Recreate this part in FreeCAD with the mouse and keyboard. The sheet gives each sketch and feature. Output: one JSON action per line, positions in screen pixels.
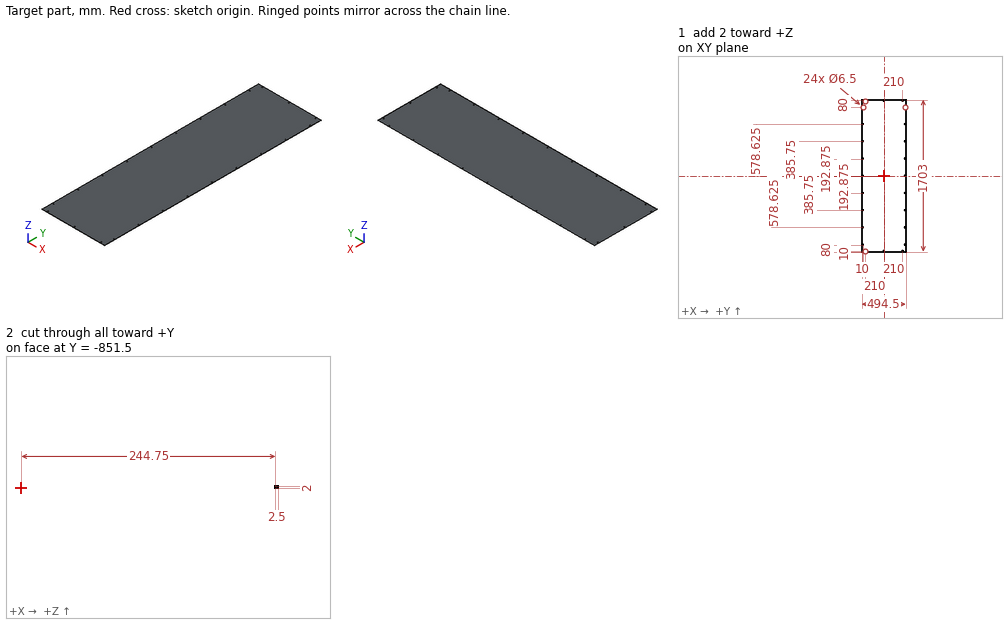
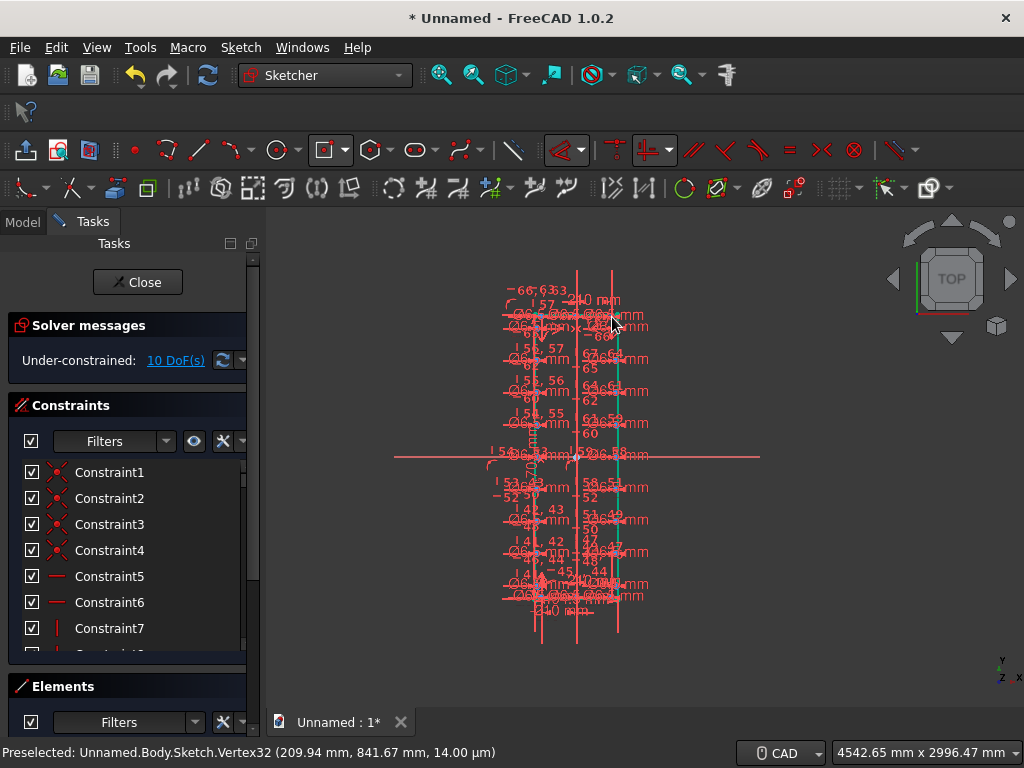
{"action": "scroll", "coordinate": [535, 599], "scroll_direction": "up", "scroll_amount": 16}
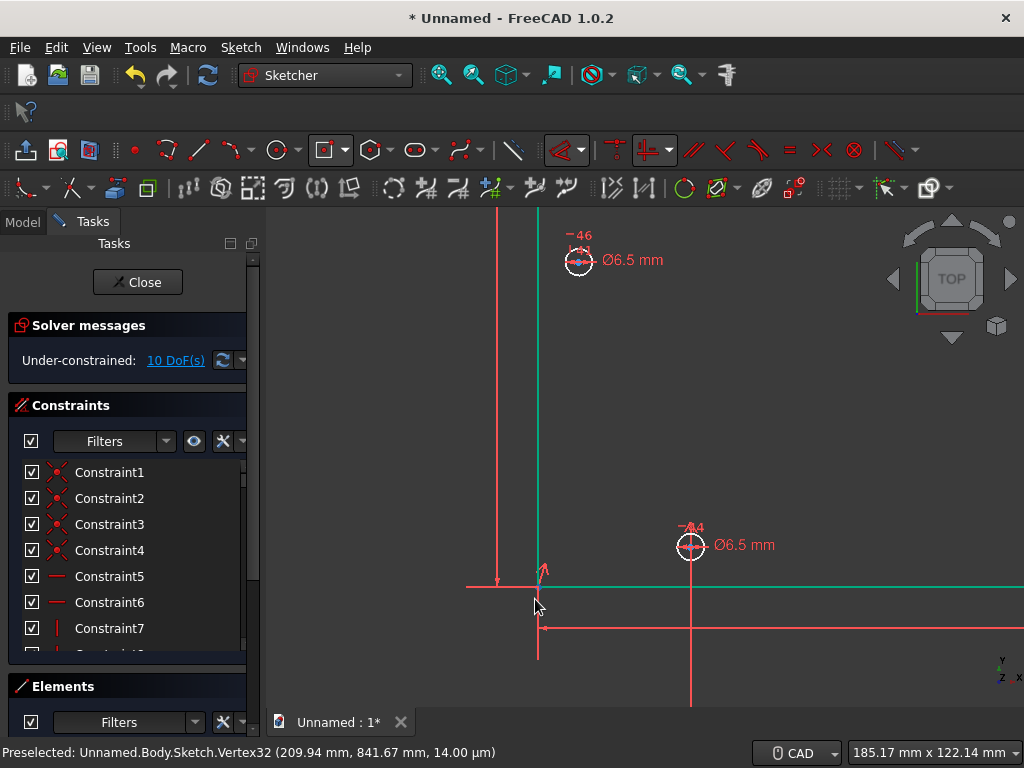
{"action": "left_click", "coordinate": [538, 587]}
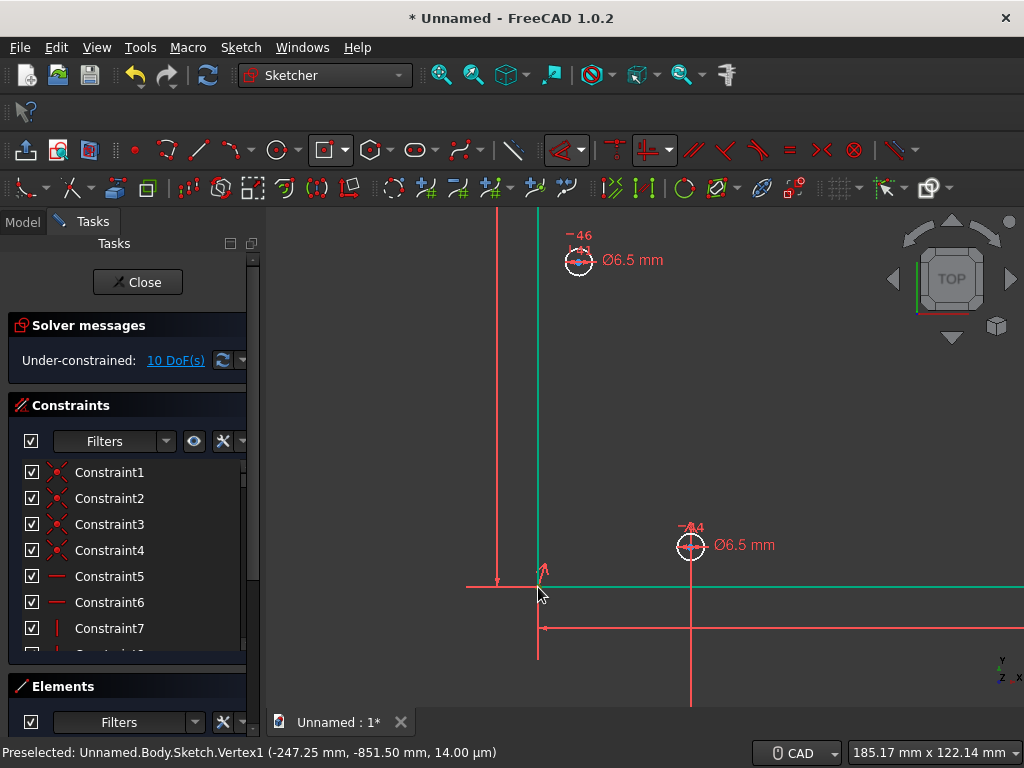
{"action": "left_click", "coordinate": [579, 262]}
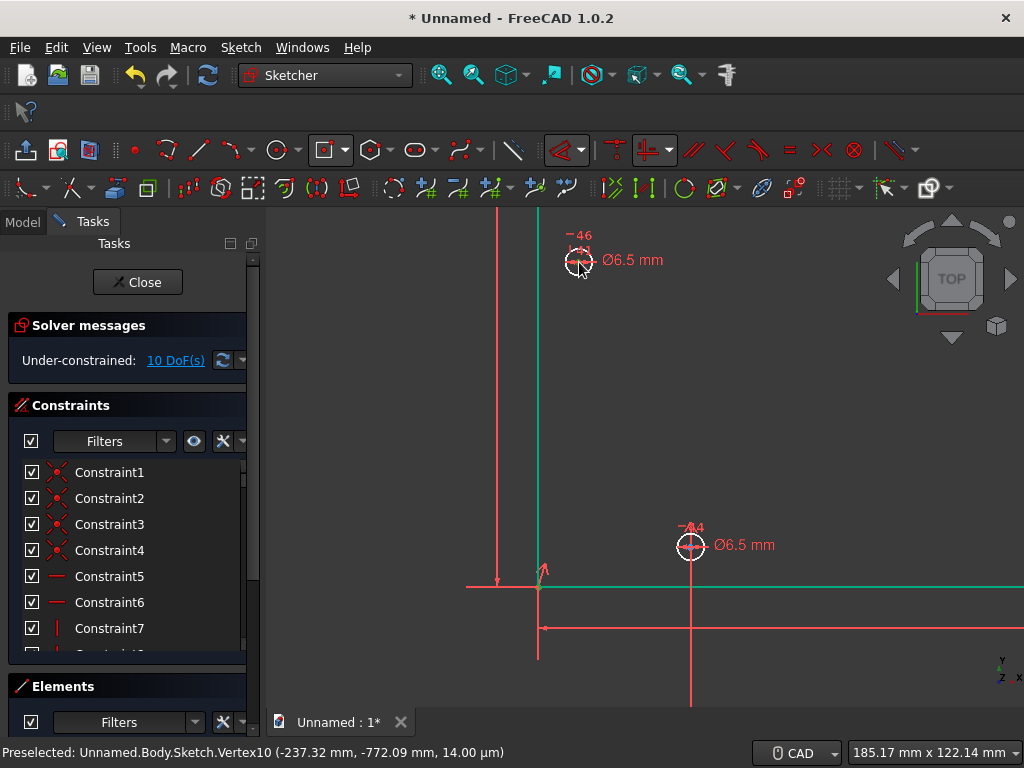
{"action": "left_click", "coordinate": [584, 150]}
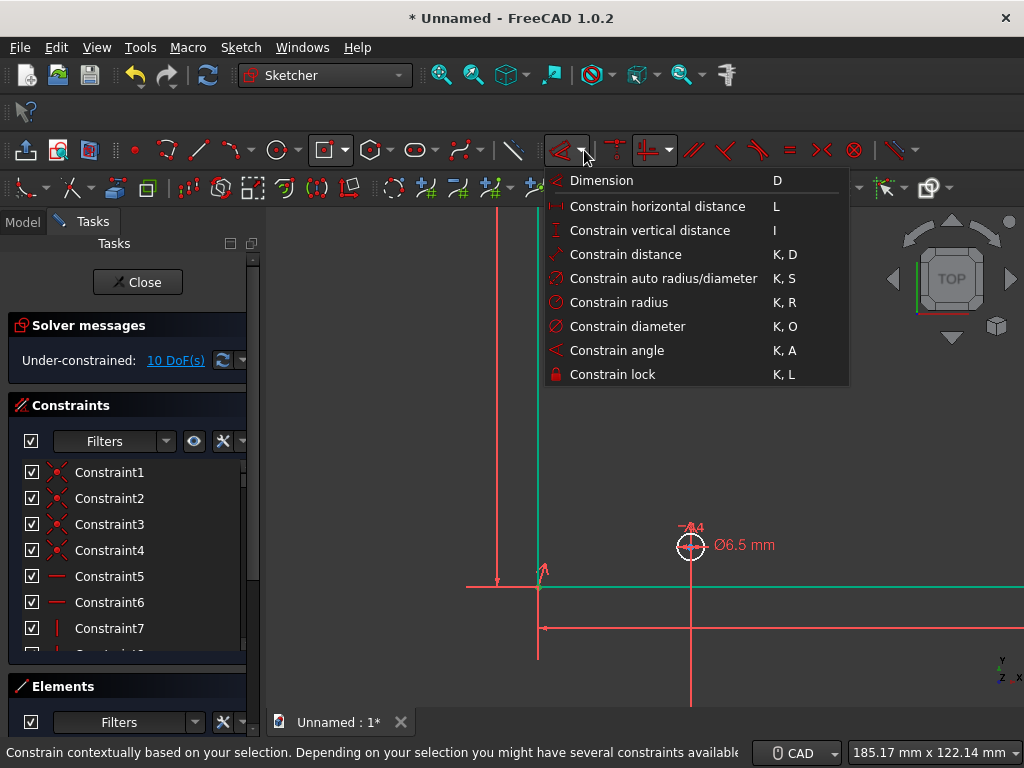
{"action": "left_click", "coordinate": [697, 206]}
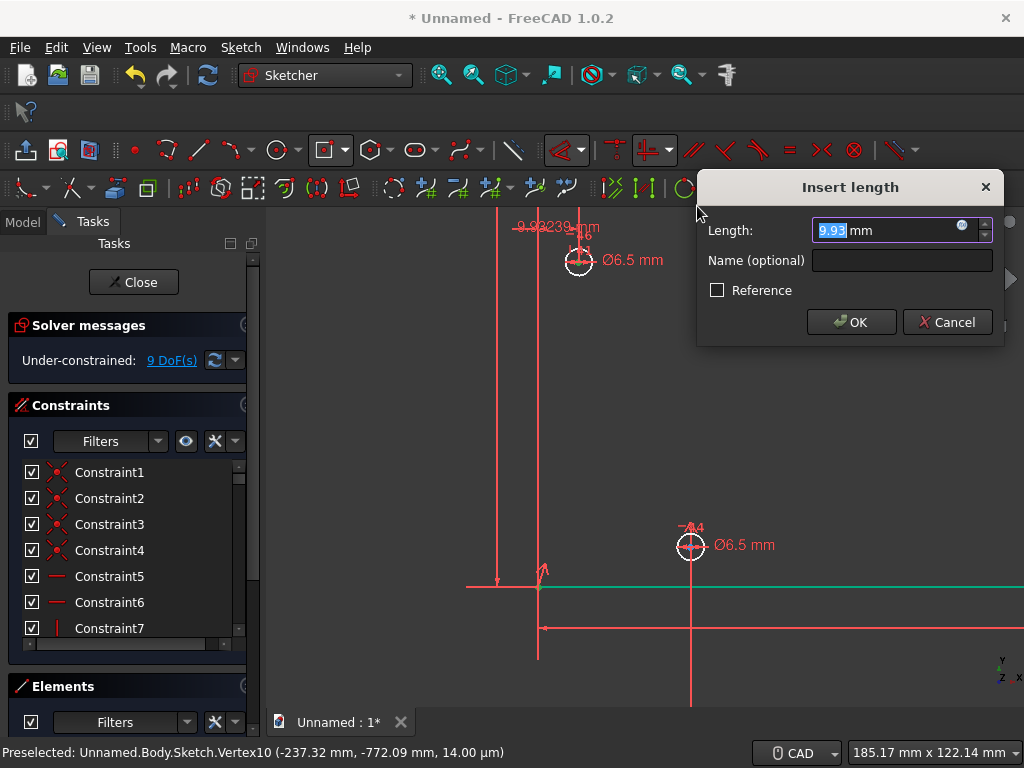
{"action": "type", "text": "10"}
{"action": "key", "text": "Return"}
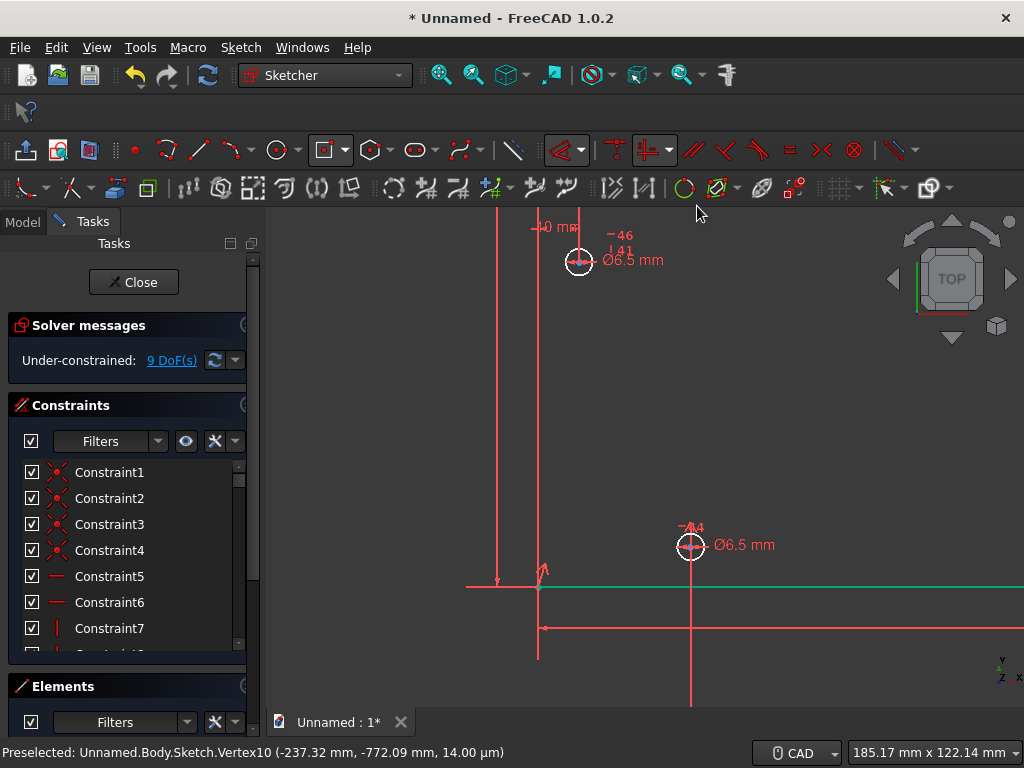
{"action": "scroll", "coordinate": [525, 633], "scroll_direction": "down", "scroll_amount": 15}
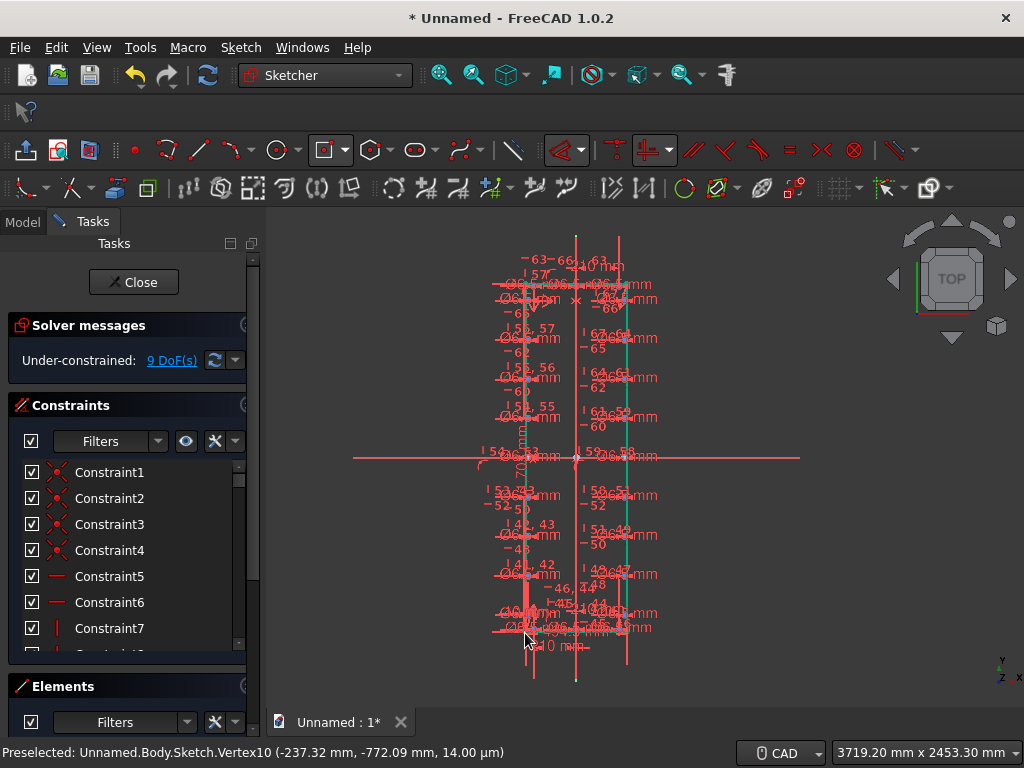
{"action": "scroll", "coordinate": [526, 632], "scroll_direction": "up", "scroll_amount": 5}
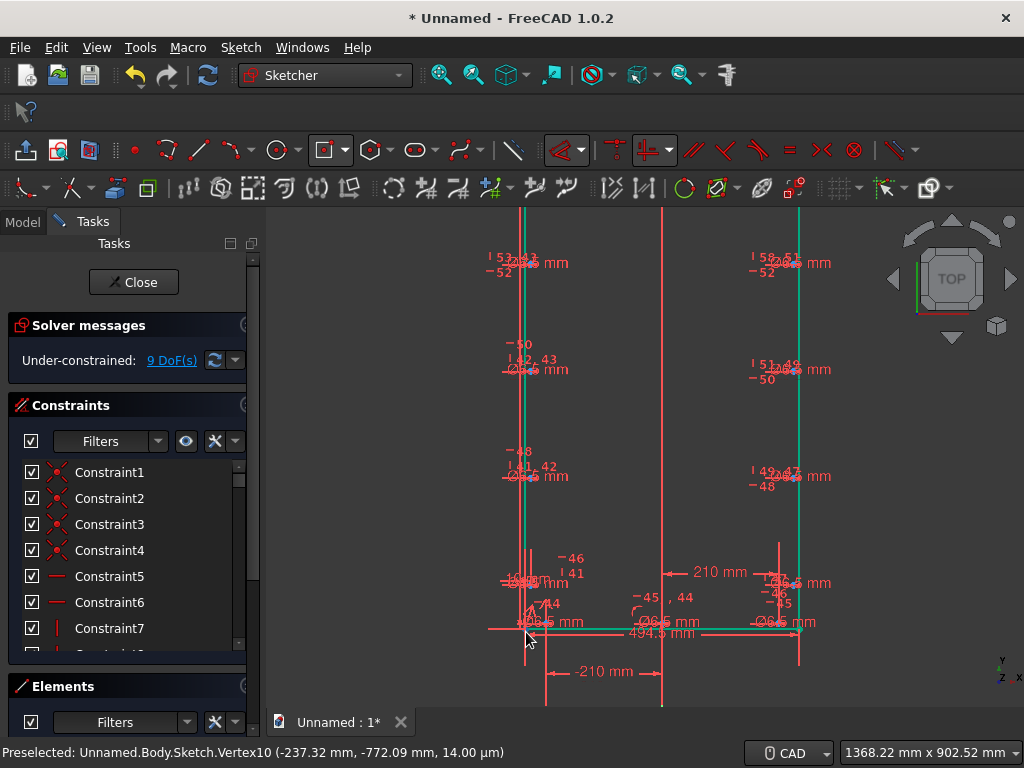
{"action": "left_click", "coordinate": [525, 629]}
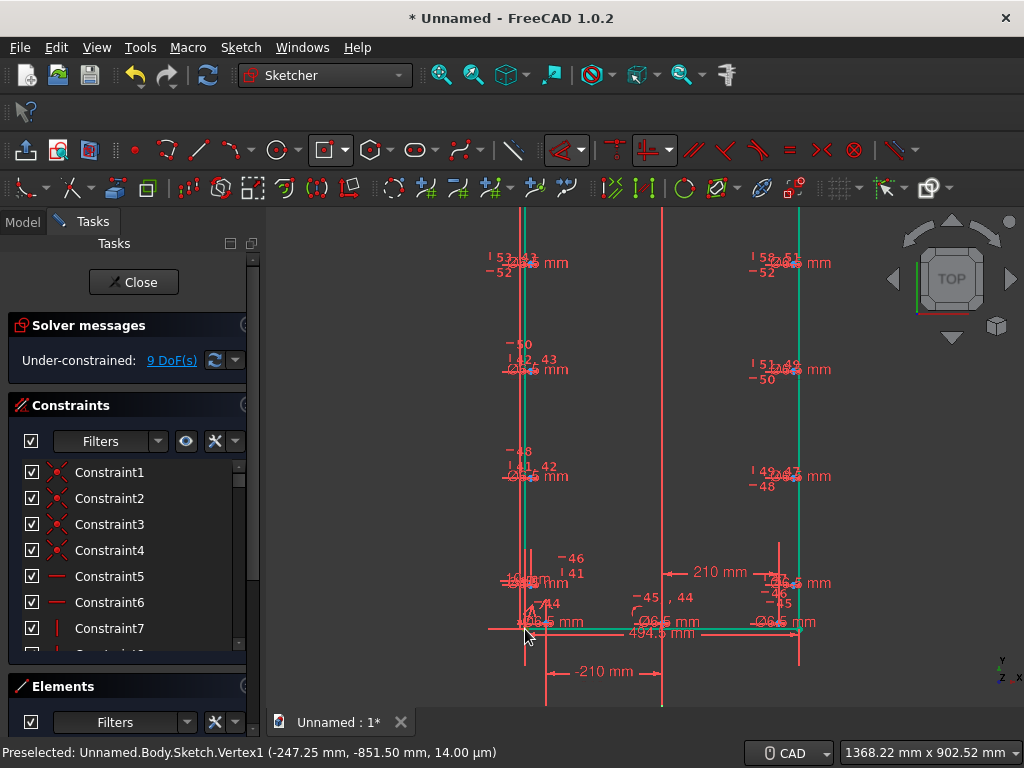
{"action": "left_click", "coordinate": [531, 585]}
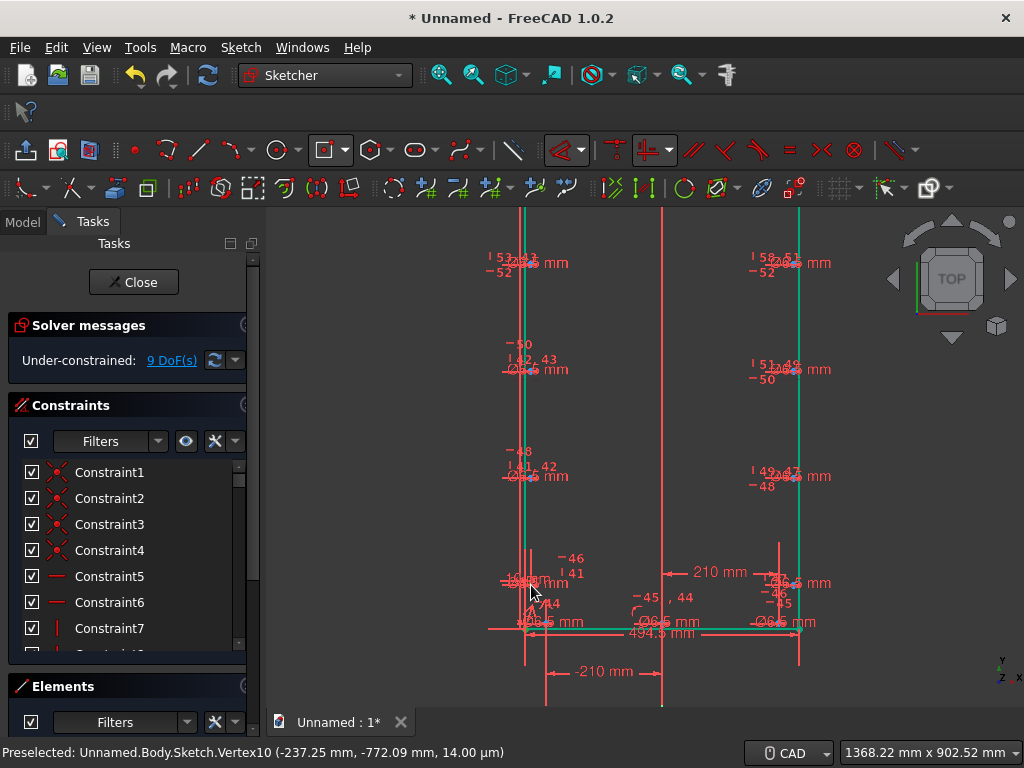
{"action": "left_click", "coordinate": [584, 150]}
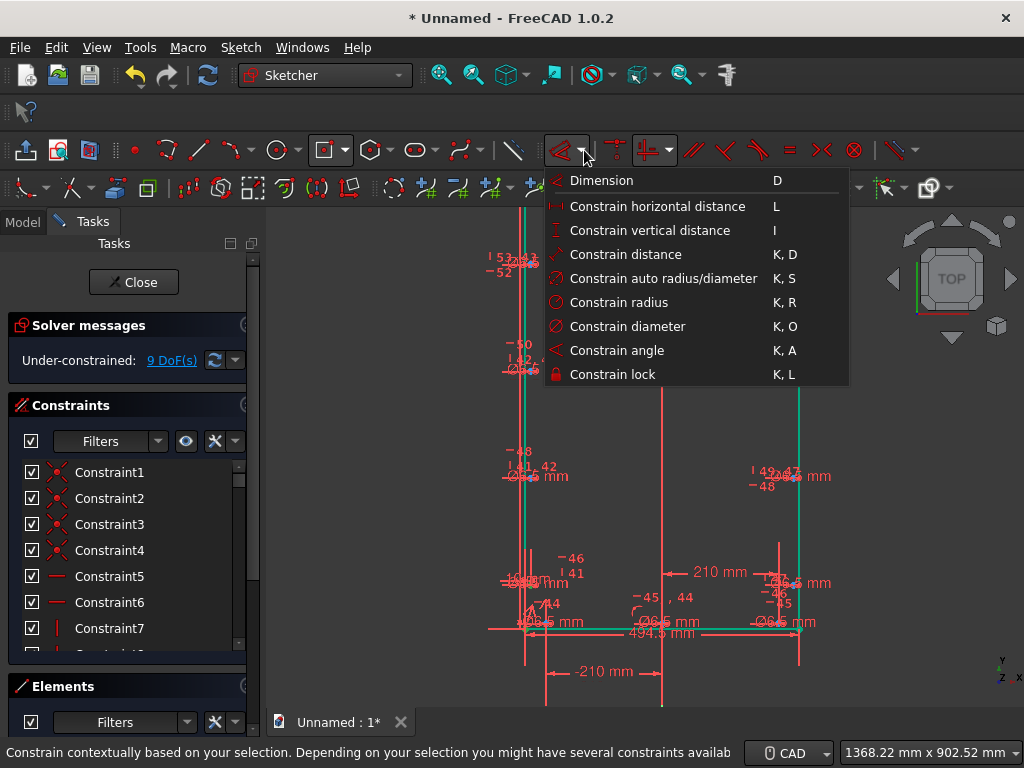
{"action": "left_click", "coordinate": [697, 230]}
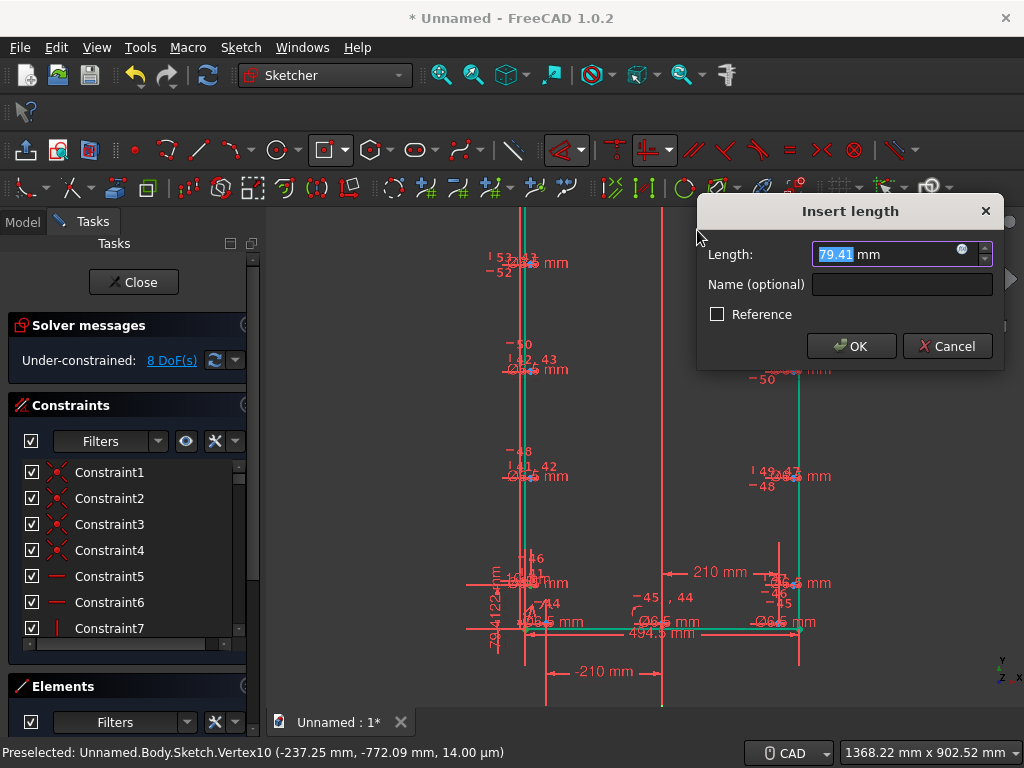
{"action": "type", "text": "80"}
{"action": "key", "text": "Return"}